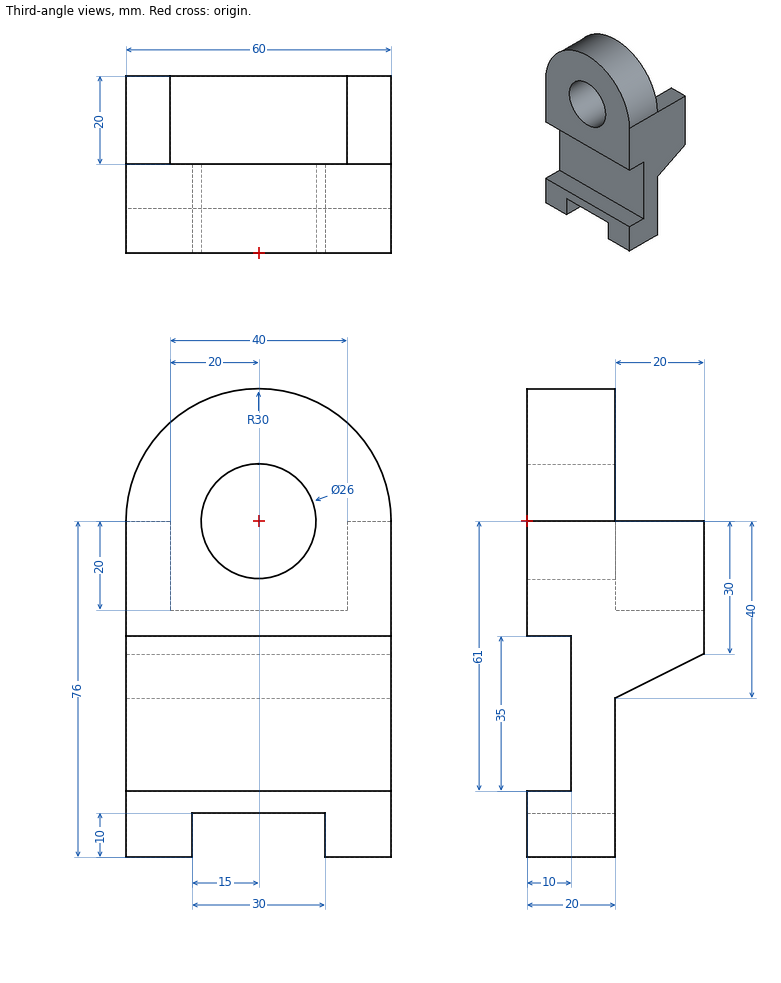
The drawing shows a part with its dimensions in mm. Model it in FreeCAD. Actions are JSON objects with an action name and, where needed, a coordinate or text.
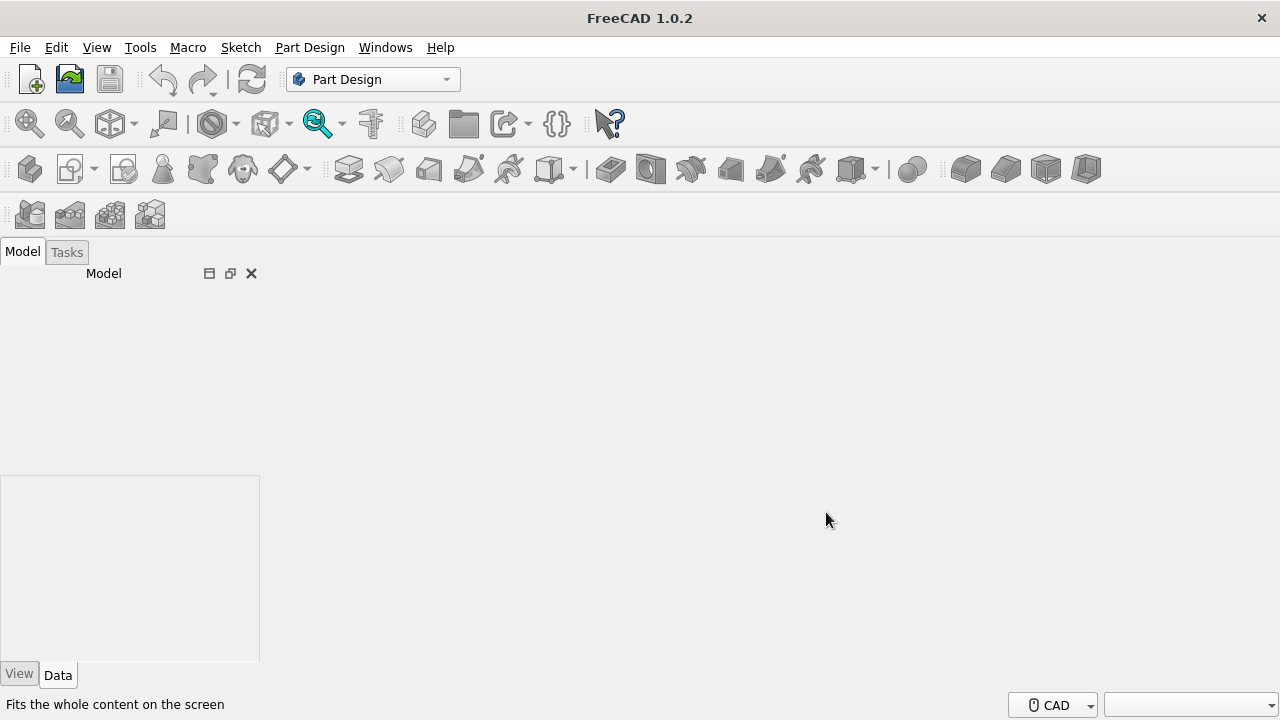
{"action": "key", "text": "ctrl+n"}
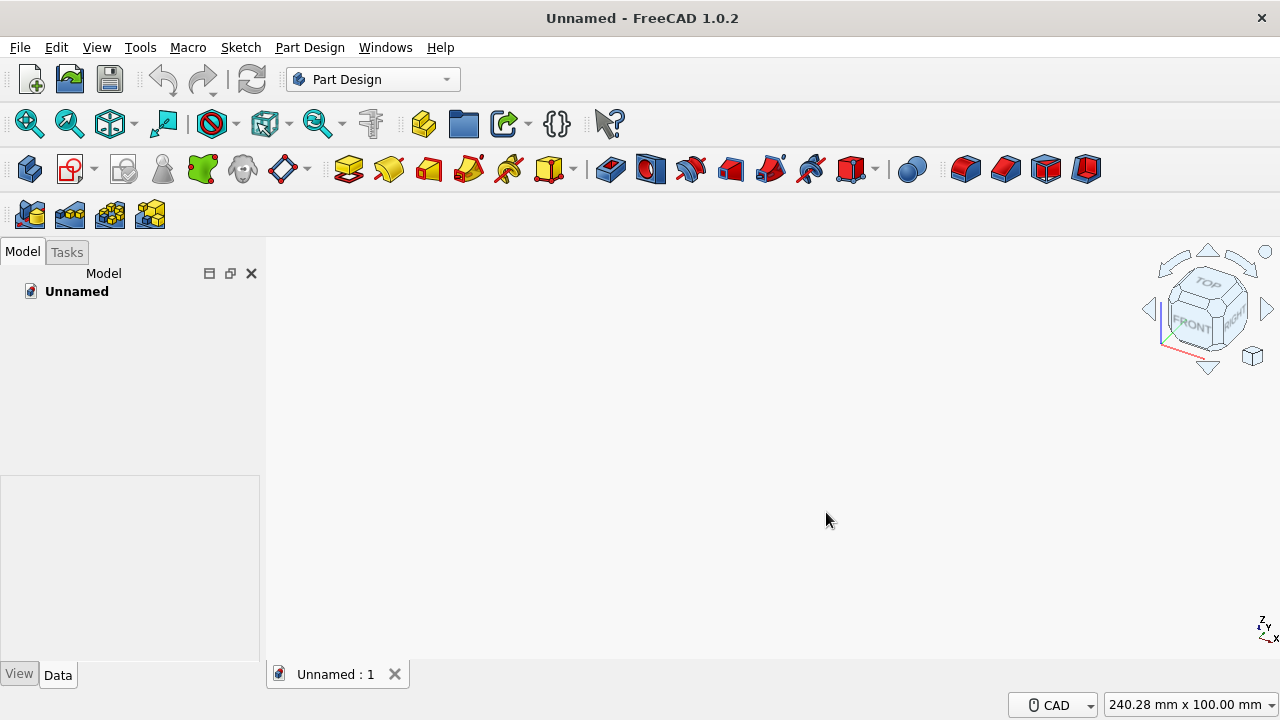
{"action": "left_click", "coordinate": [70, 170]}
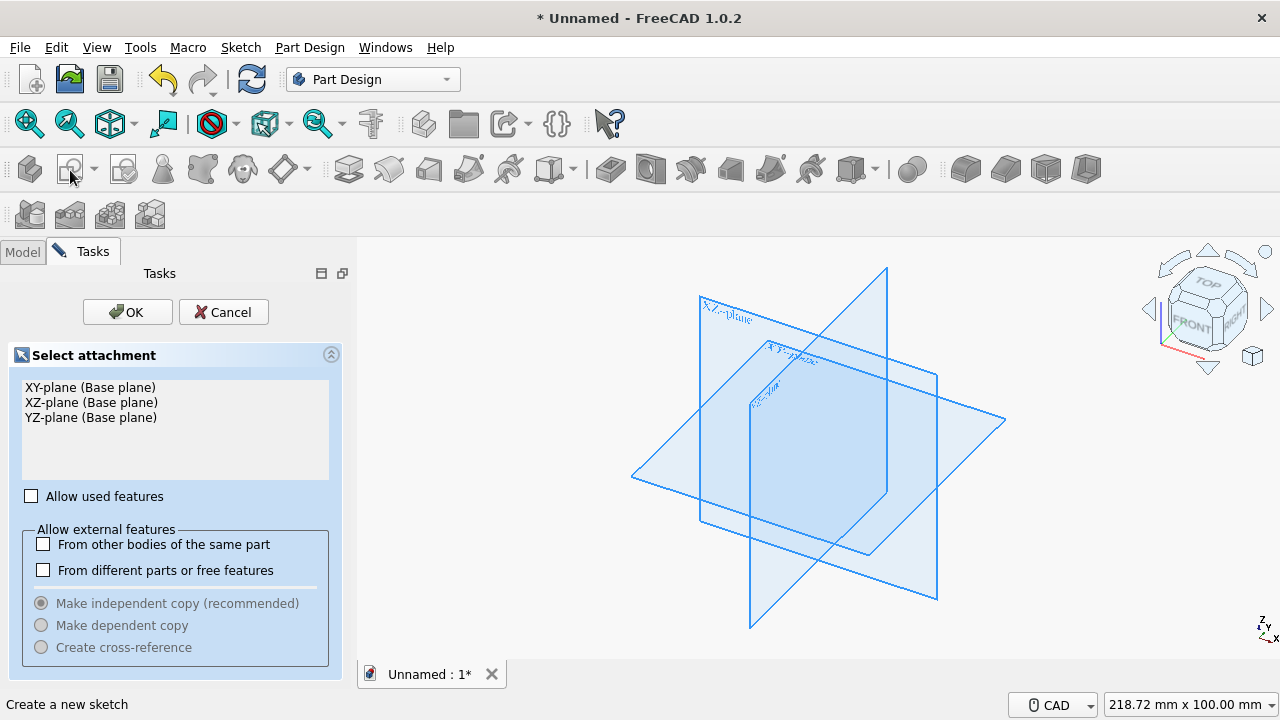
{"action": "left_click", "coordinate": [82, 402]}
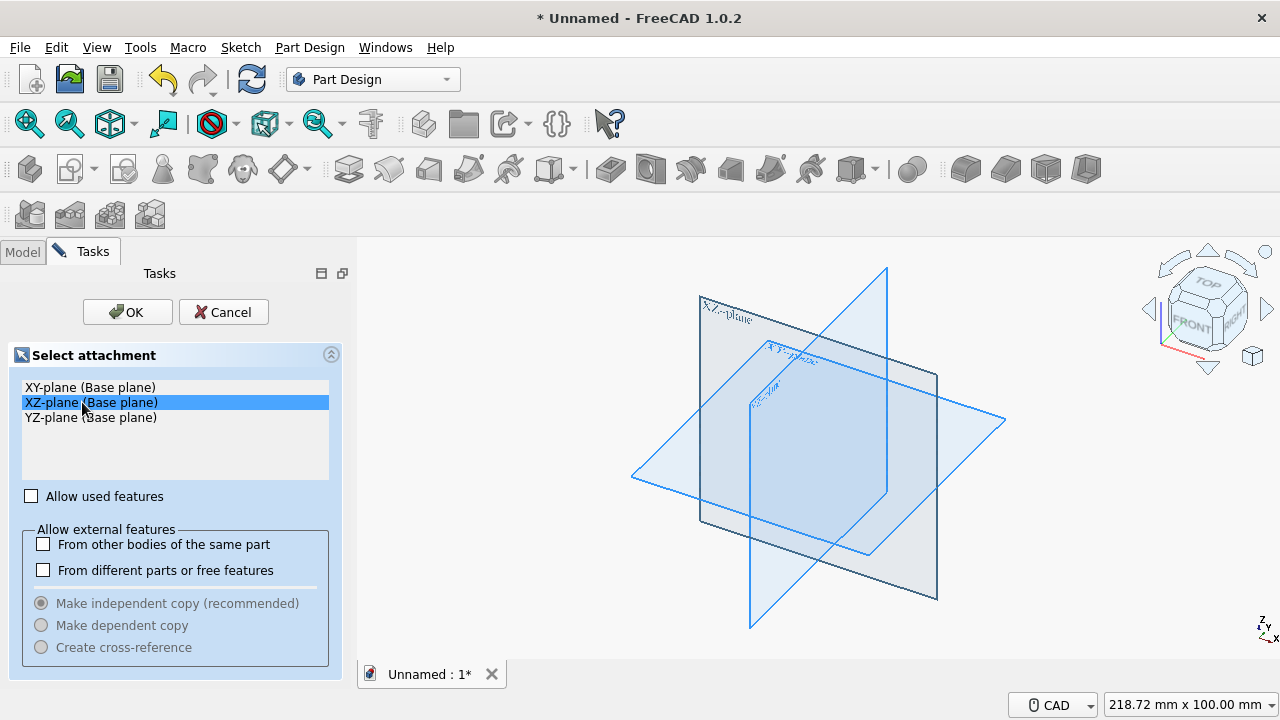
{"action": "left_click", "coordinate": [128, 312]}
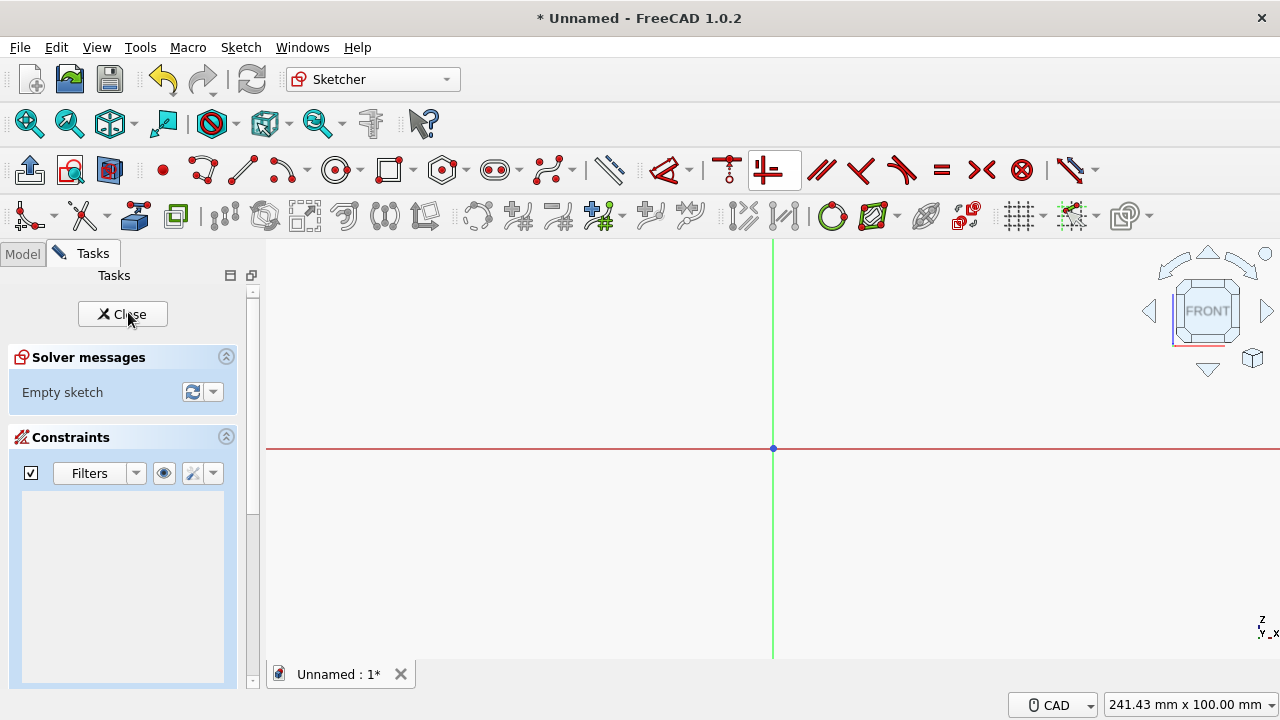
{"action": "scroll", "coordinate": [621, 331], "scroll_direction": "down", "scroll_amount": 3}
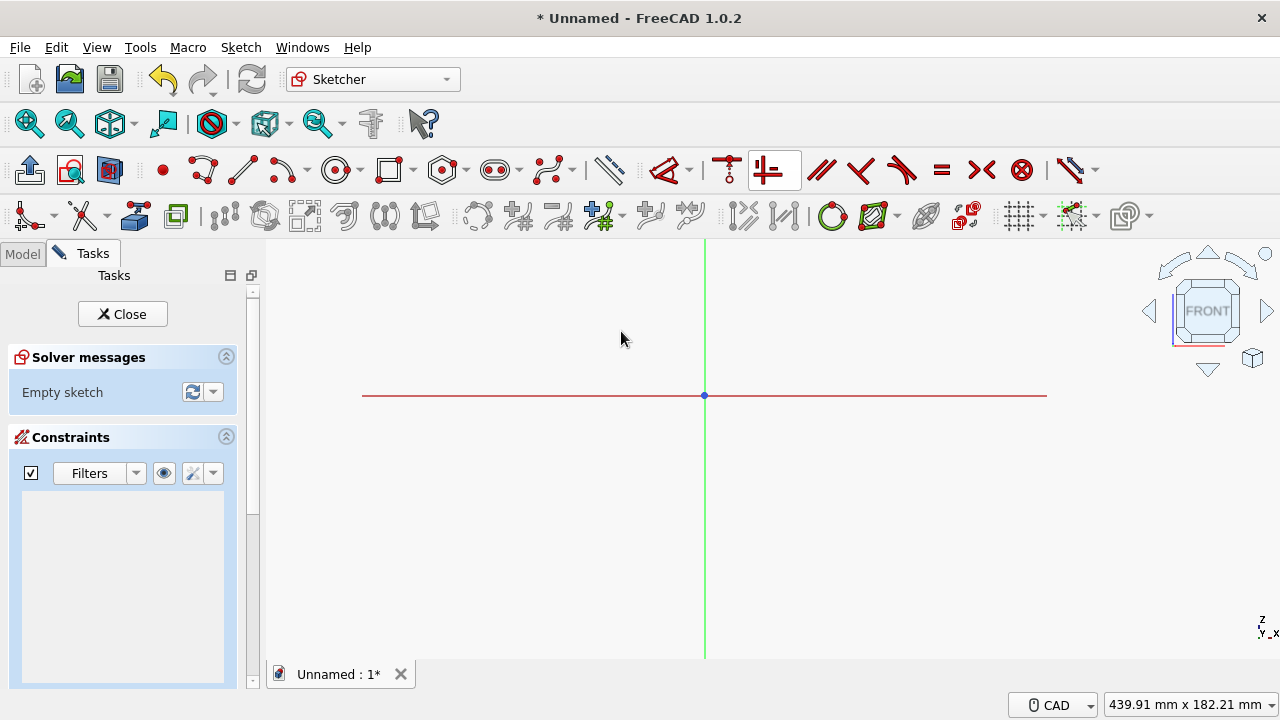
{"action": "left_click", "coordinate": [204, 170]}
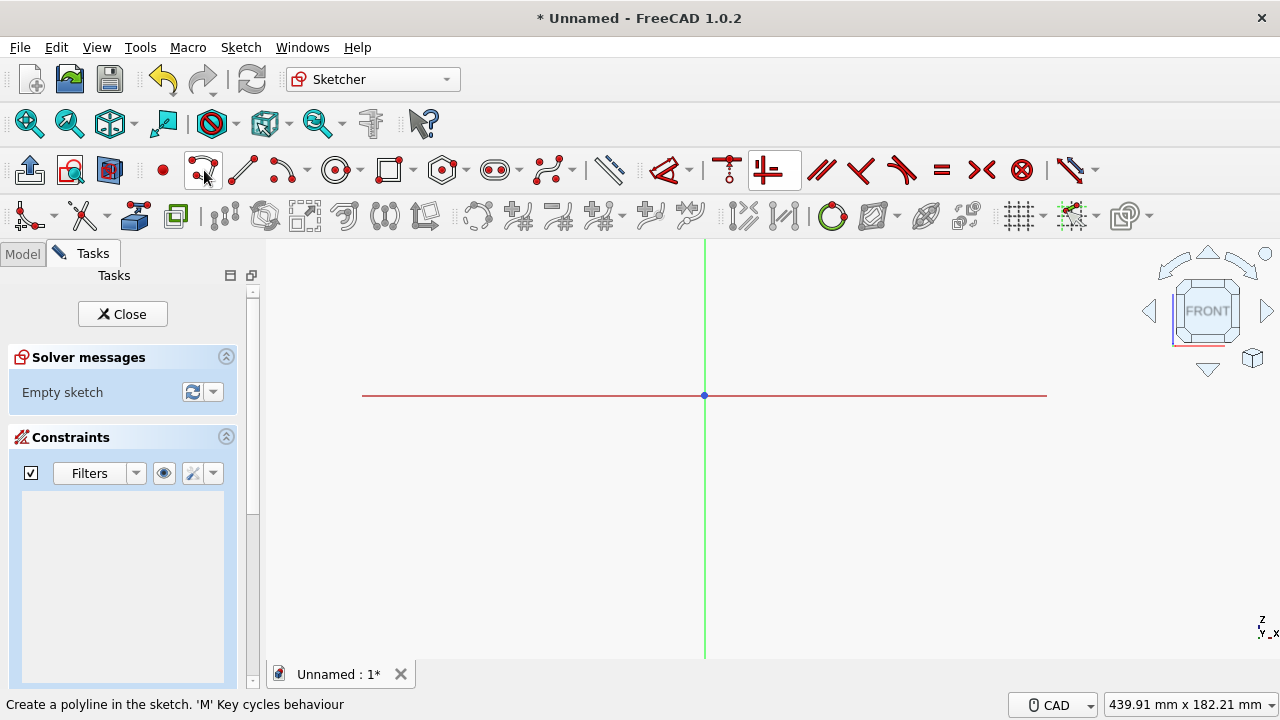
{"action": "left_click", "coordinate": [635, 396]}
{"action": "left_click", "coordinate": [635, 571]}
{"action": "left_click", "coordinate": [774, 571]}
{"action": "left_click", "coordinate": [774, 396]}
{"action": "right_click", "coordinate": [774, 396]}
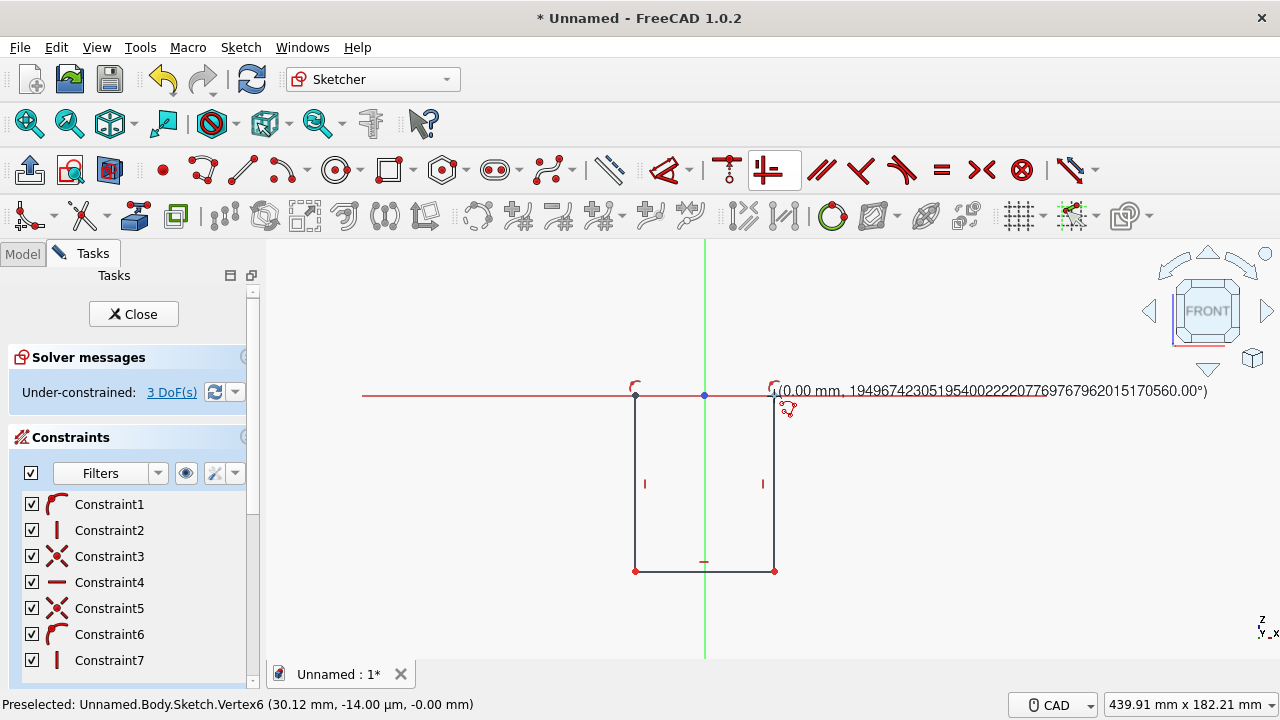
{"action": "key", "text": "g 3 a"}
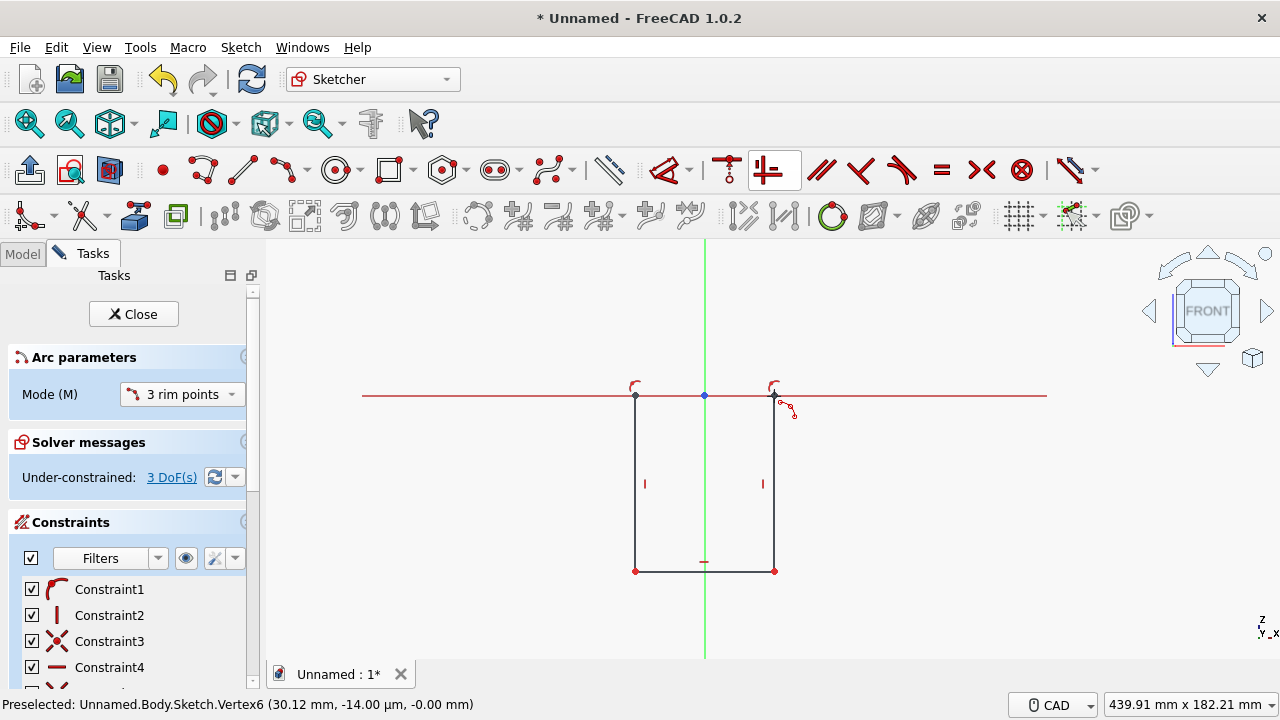
{"action": "left_click", "coordinate": [774, 396]}
{"action": "left_click", "coordinate": [635, 396]}
{"action": "left_click", "coordinate": [726, 330]}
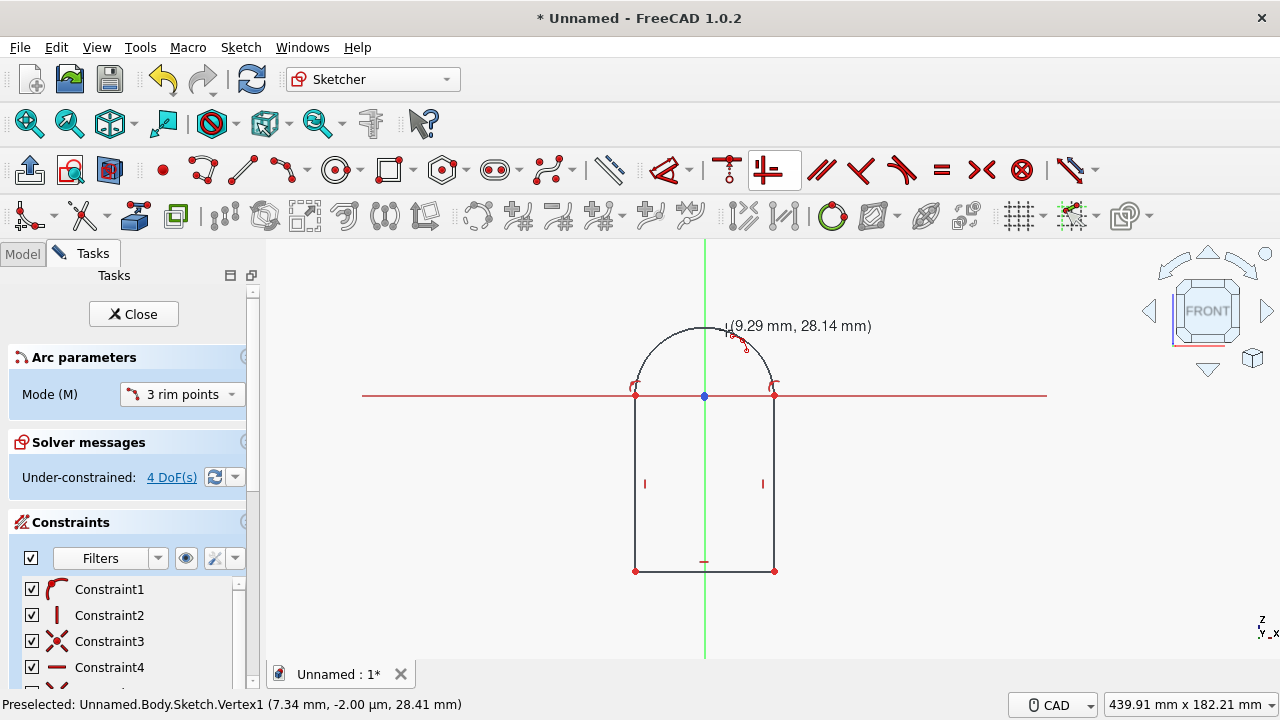
{"action": "key", "text": "g c"}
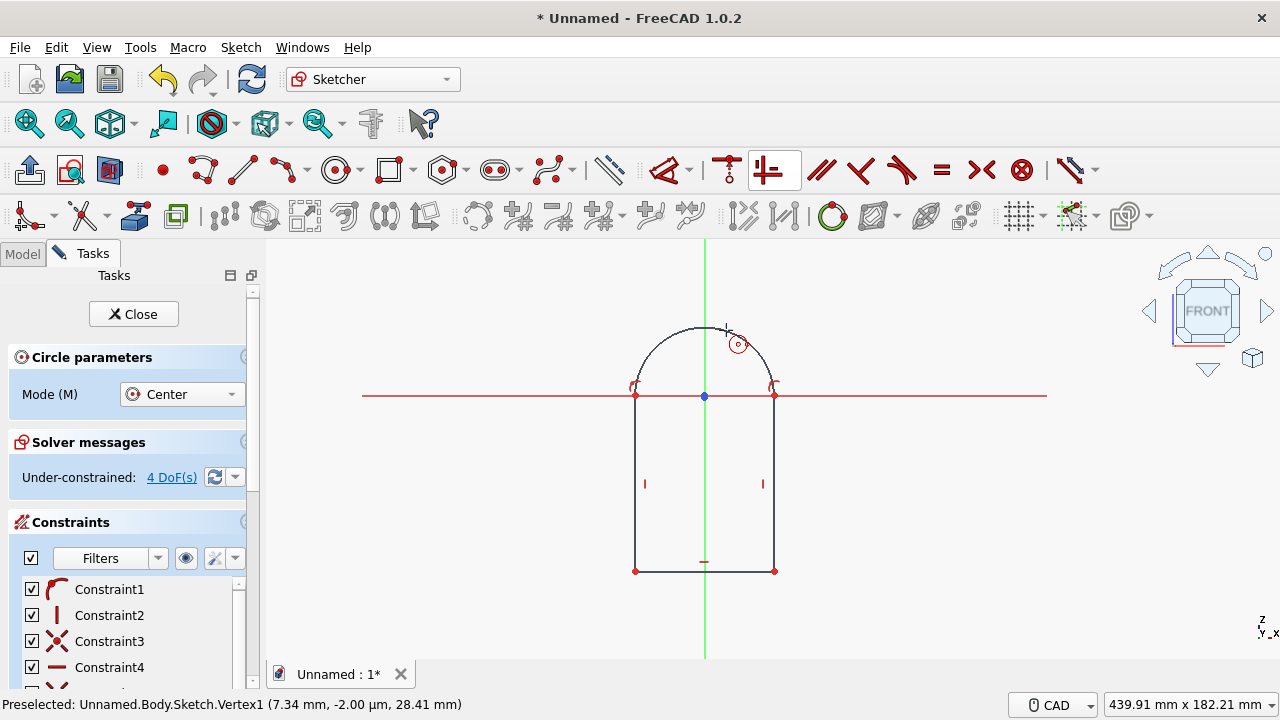
{"action": "left_click", "coordinate": [705, 396]}
{"action": "left_click", "coordinate": [726, 375]}
{"action": "key", "text": "Escape"}